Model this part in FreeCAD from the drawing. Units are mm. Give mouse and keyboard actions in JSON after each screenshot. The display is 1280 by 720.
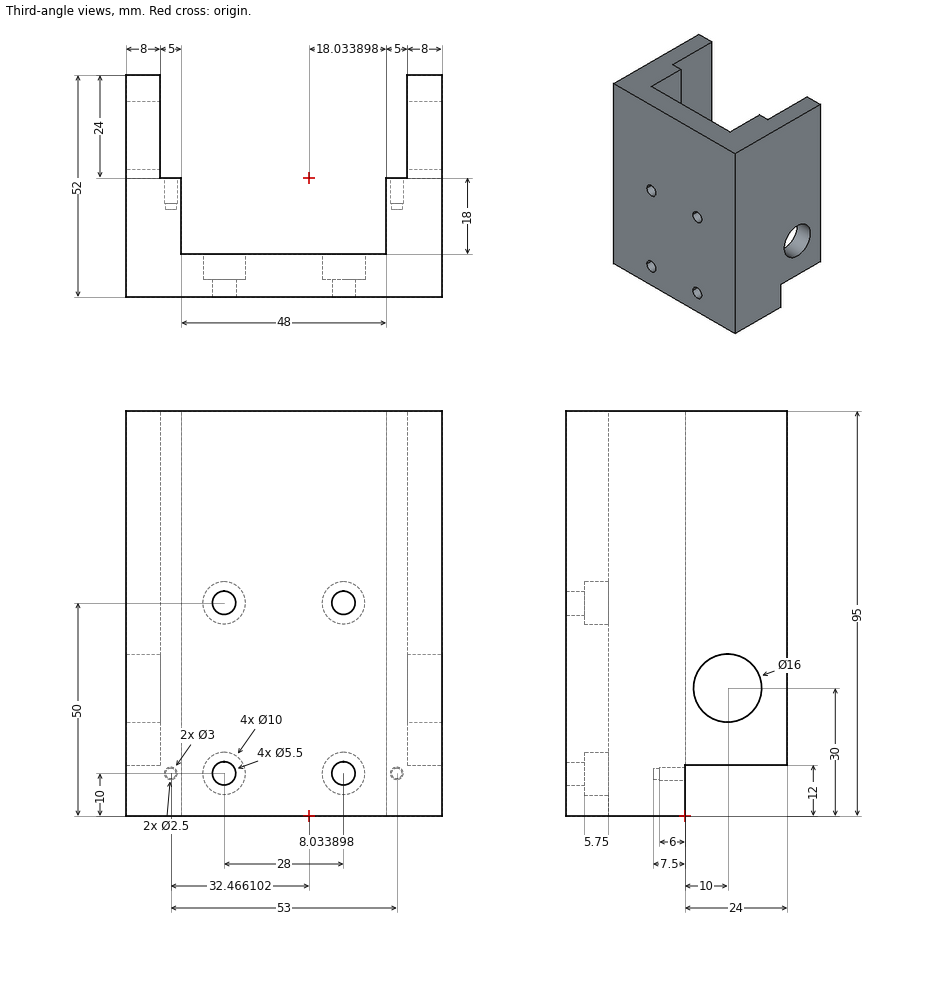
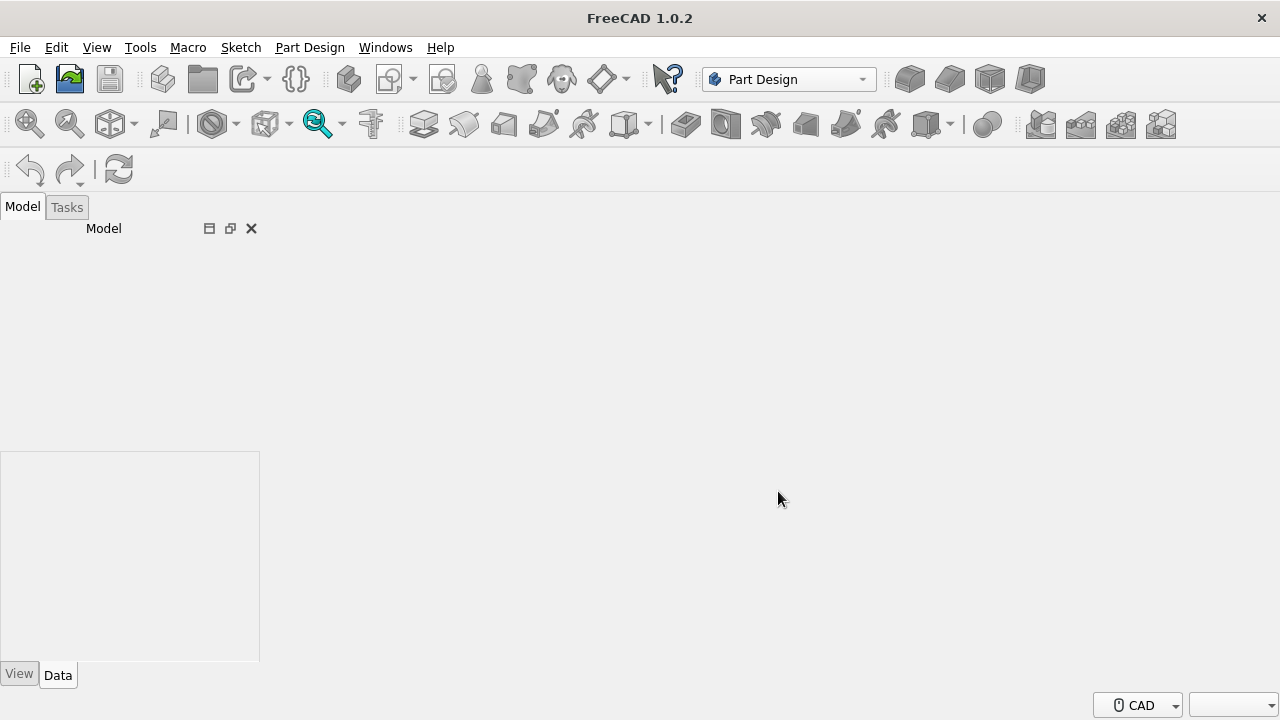
{"action": "key", "text": "ctrl+n"}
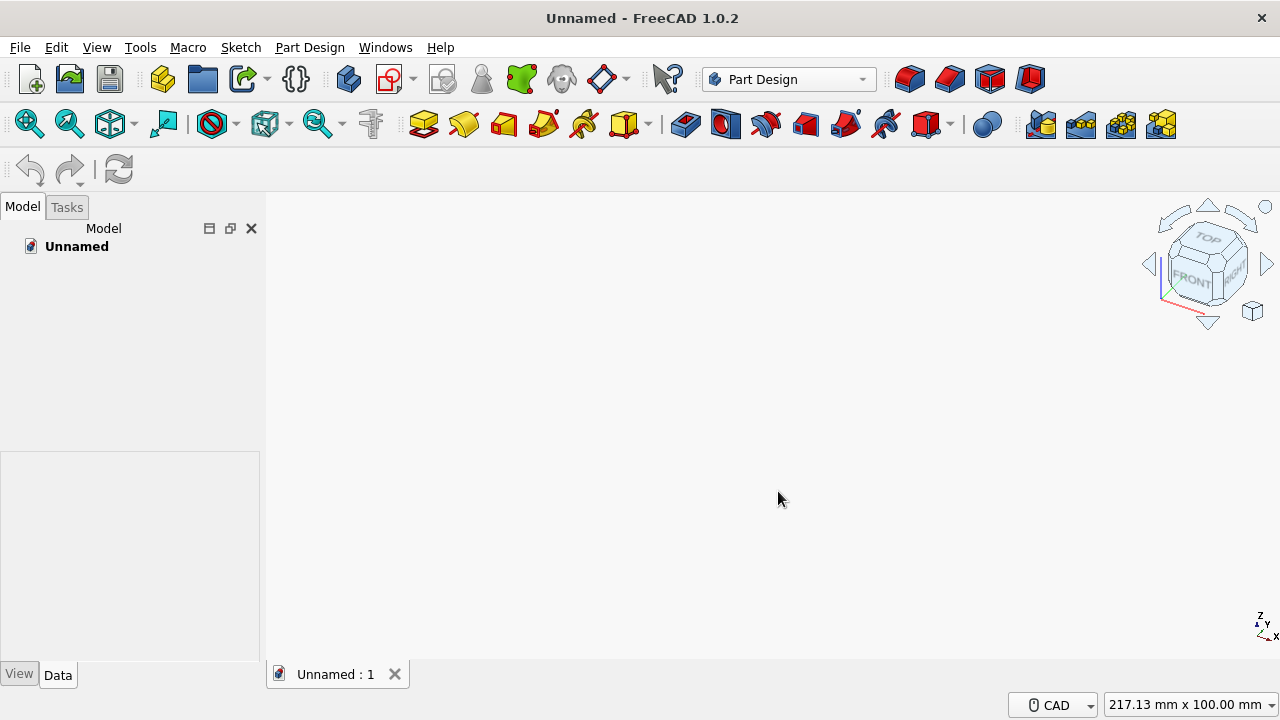
{"action": "left_click", "coordinate": [390, 80]}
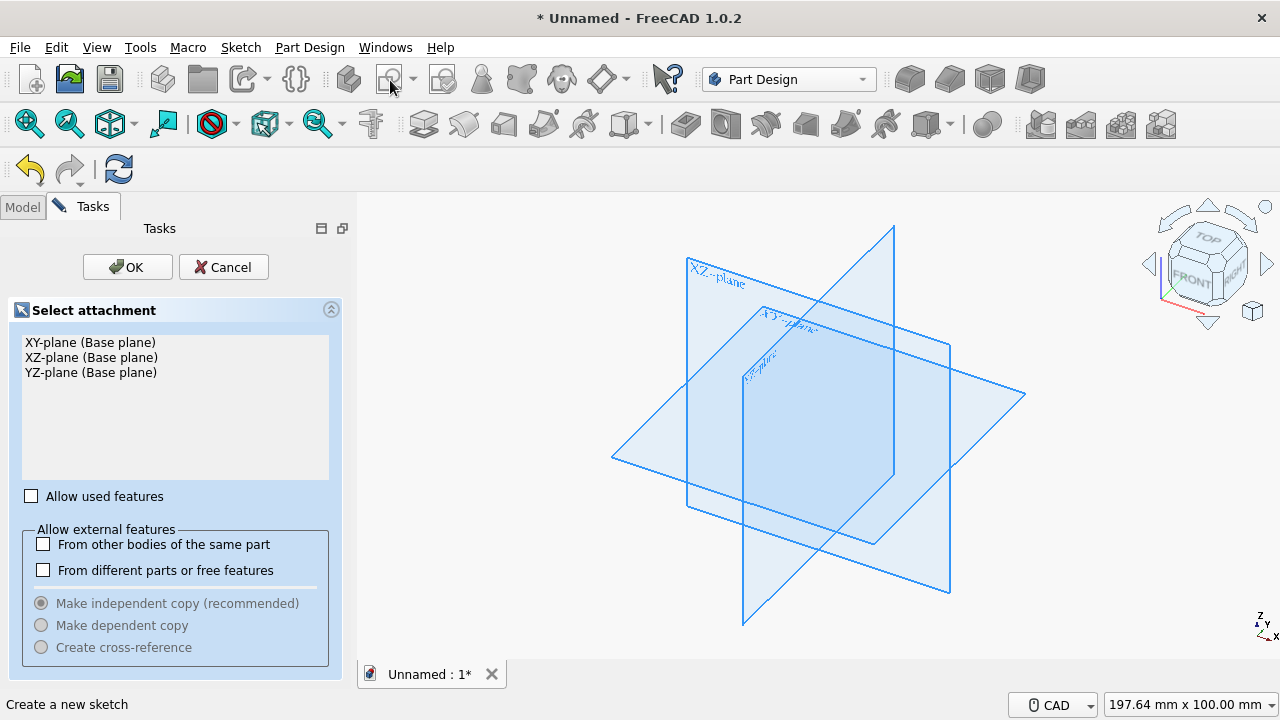
{"action": "left_click", "coordinate": [82, 342]}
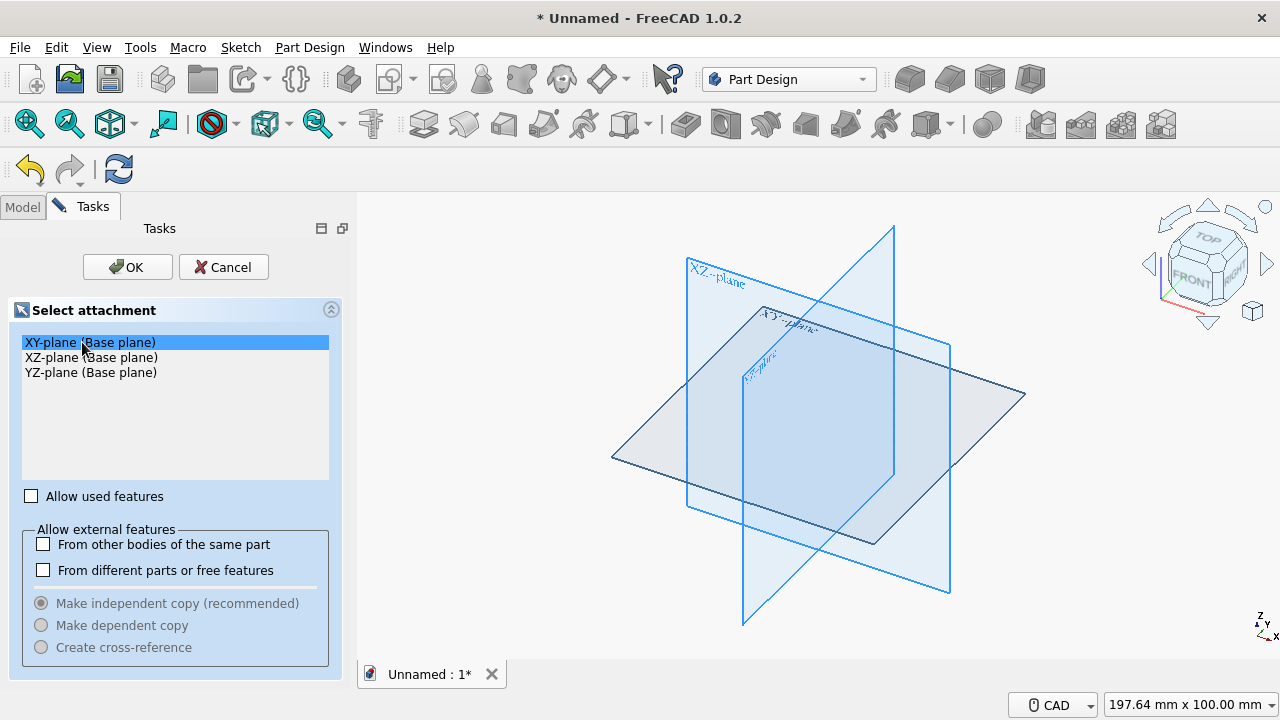
{"action": "left_click", "coordinate": [128, 267]}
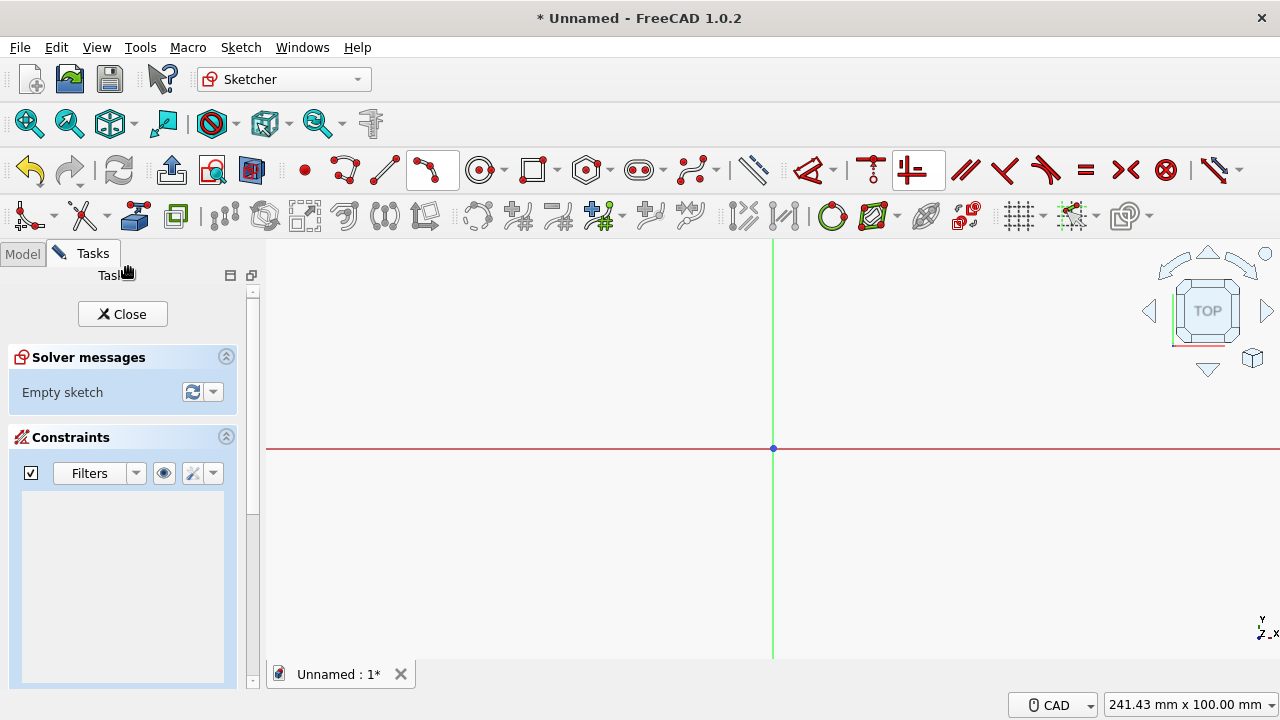
{"action": "left_click", "coordinate": [346, 170]}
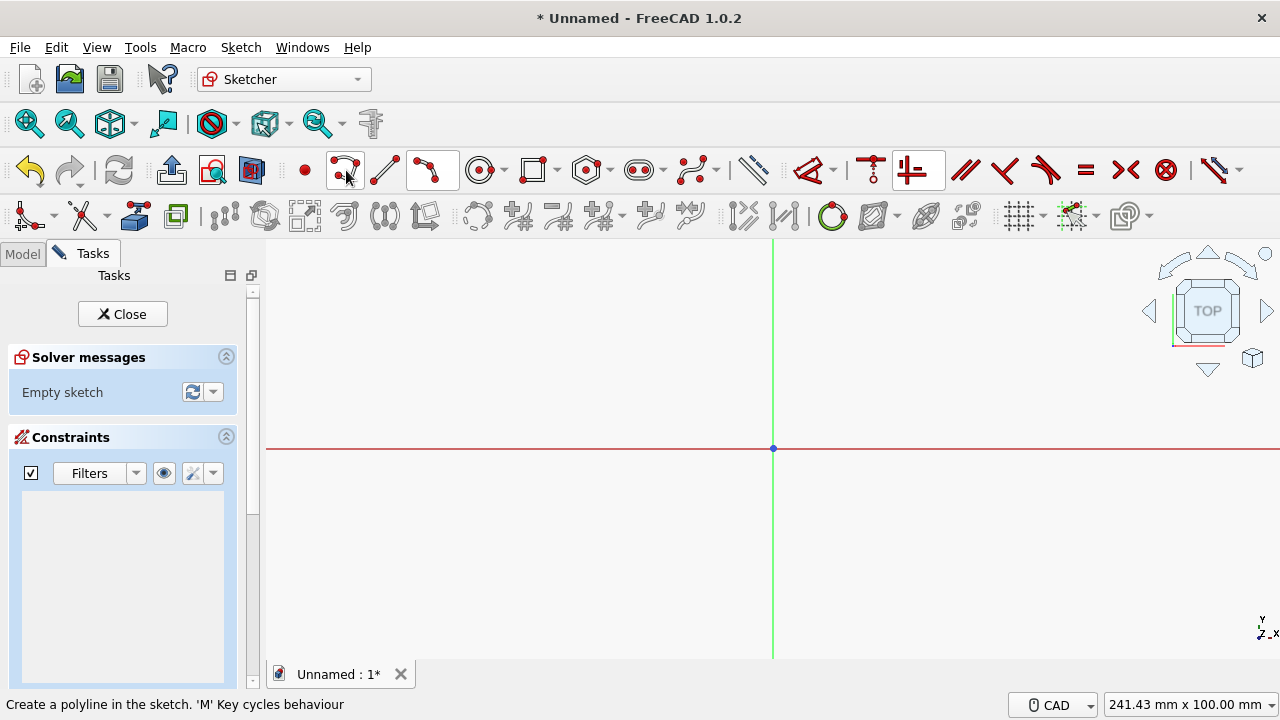
{"action": "left_click", "coordinate": [849, 449]}
{"action": "left_click", "coordinate": [849, 525]}
{"action": "left_click", "coordinate": [647, 525]}
{"action": "left_click", "coordinate": [647, 449]}
{"action": "left_click", "coordinate": [626, 458]}
{"action": "left_click", "coordinate": [626, 348]}
{"action": "left_click", "coordinate": [593, 348]}
{"action": "left_click", "coordinate": [593, 567]}
{"action": "left_click", "coordinate": [903, 567]}
{"action": "left_click", "coordinate": [903, 348]}
{"action": "left_click", "coordinate": [870, 348]}
{"action": "left_click", "coordinate": [870, 458]}
{"action": "left_click", "coordinate": [849, 449]}
{"action": "key", "text": "Escape"}
{"action": "key", "text": "Escape"}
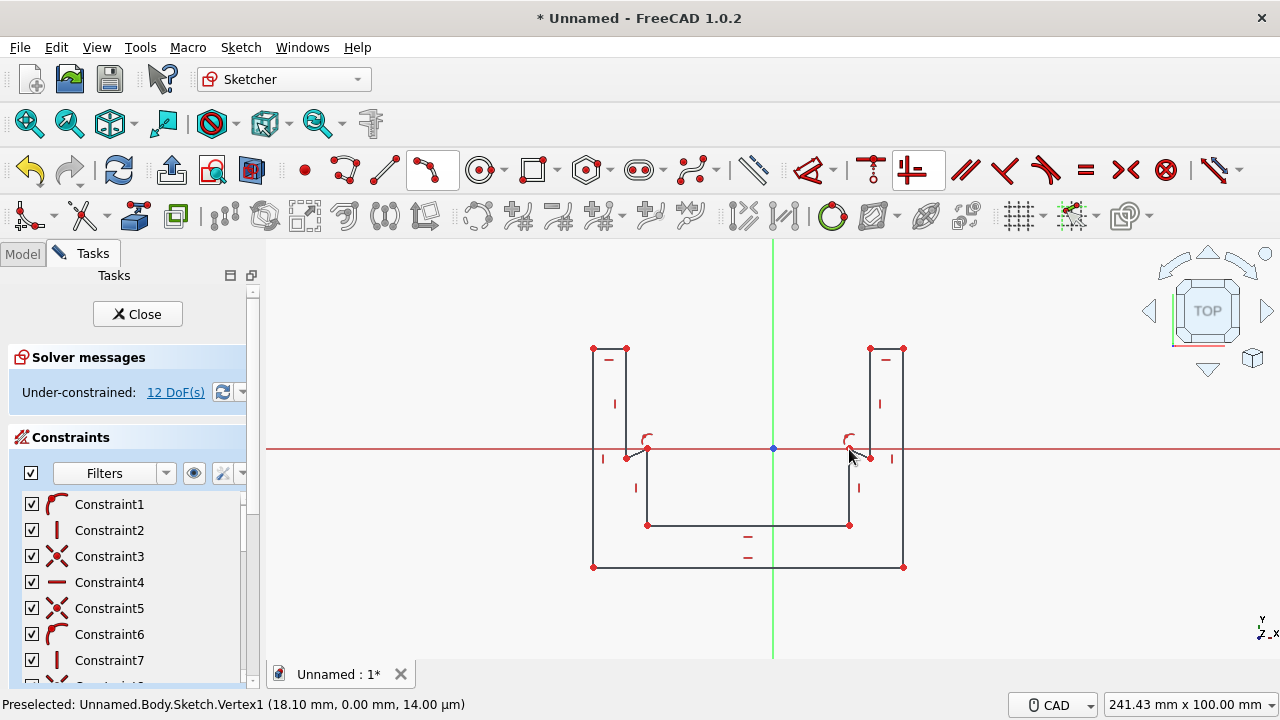
{"action": "scroll", "coordinate": [639, 453], "scroll_direction": "up", "scroll_amount": 3}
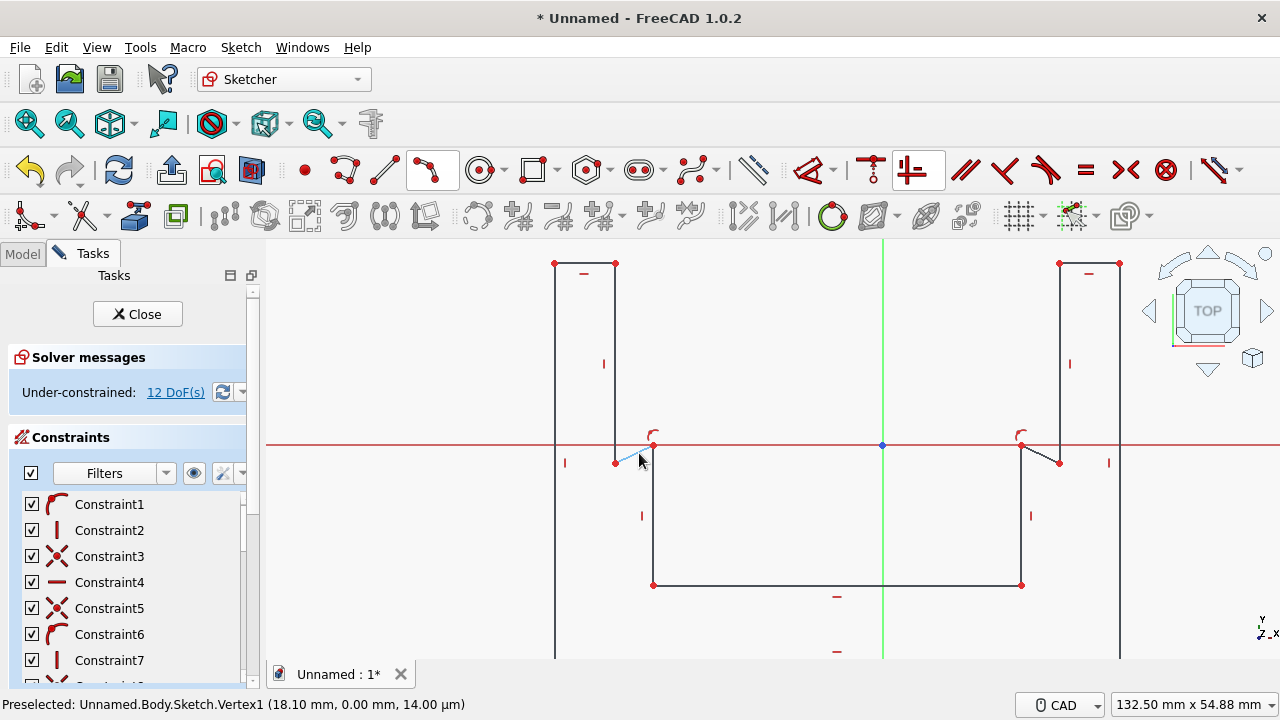
{"action": "left_click", "coordinate": [638, 453]}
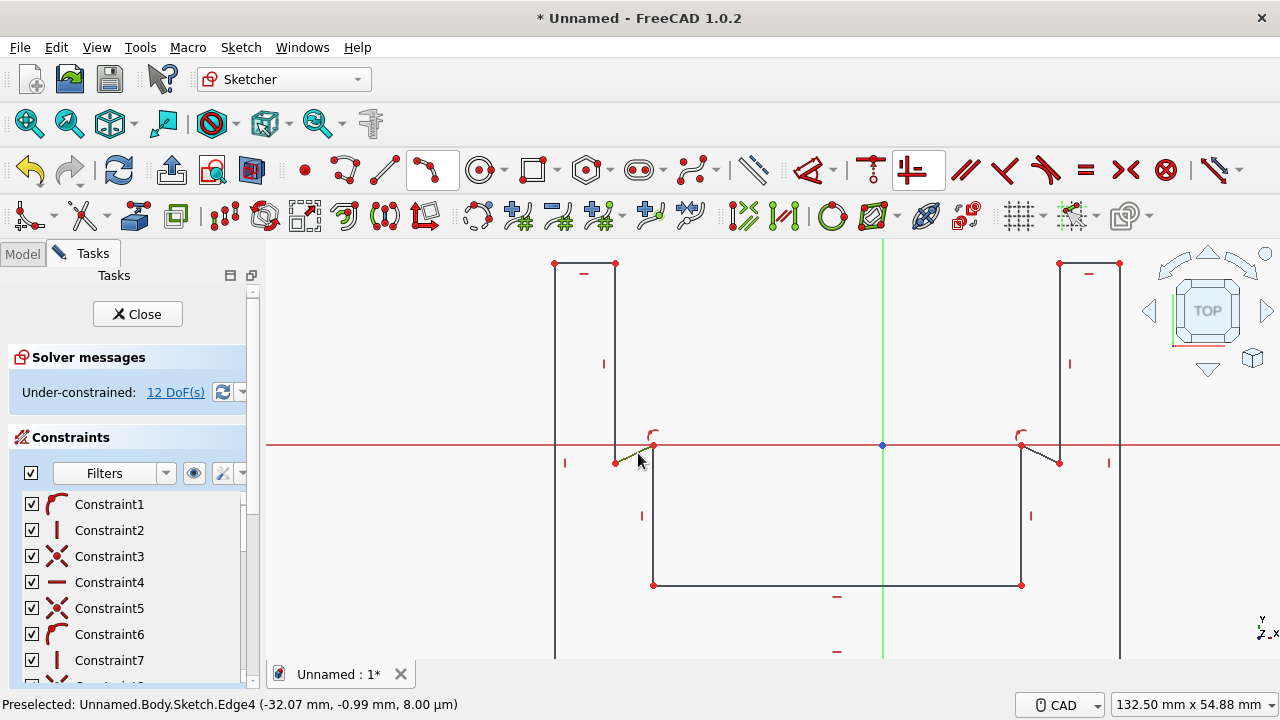
{"action": "key", "text": "h"}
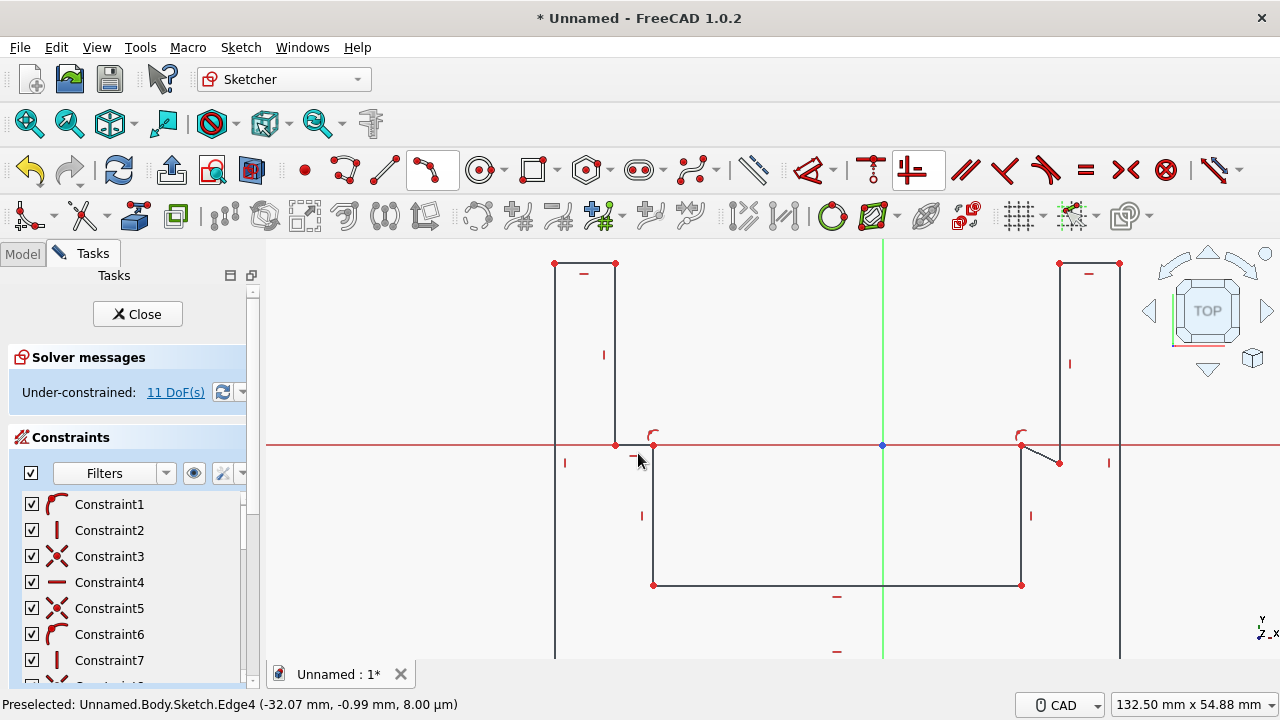
{"action": "left_click", "coordinate": [1048, 458]}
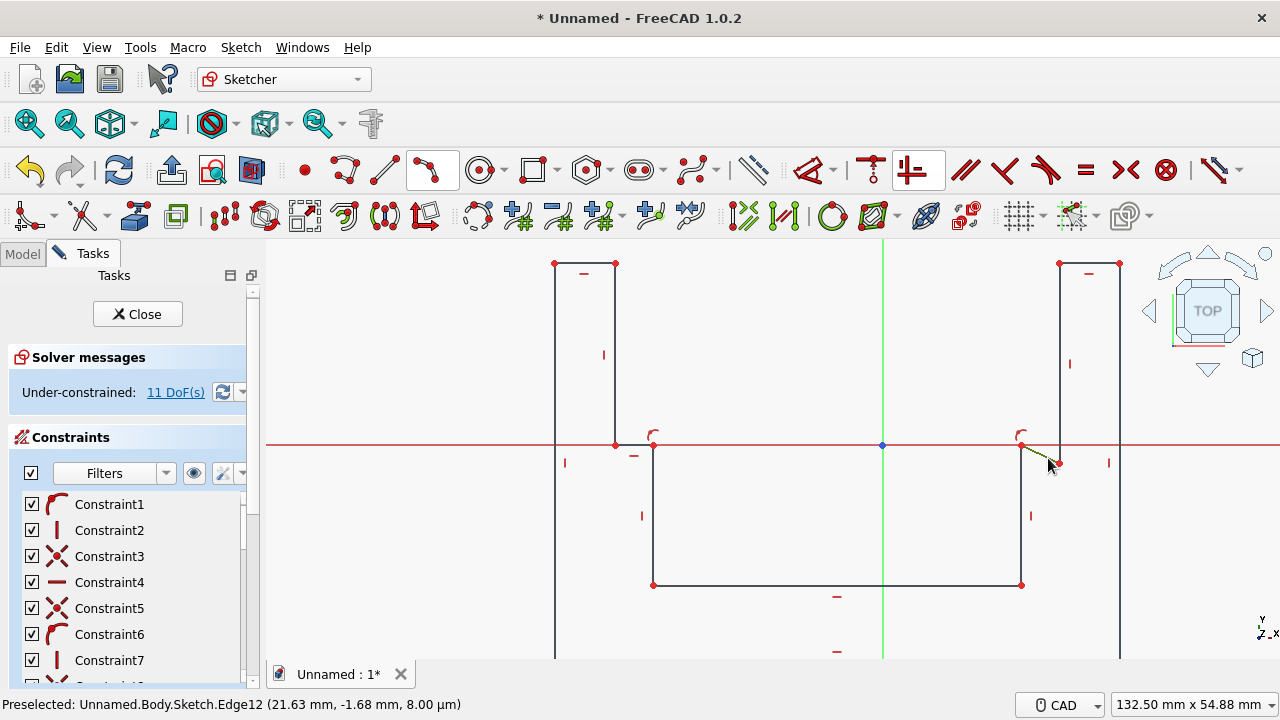
{"action": "key", "text": "h"}